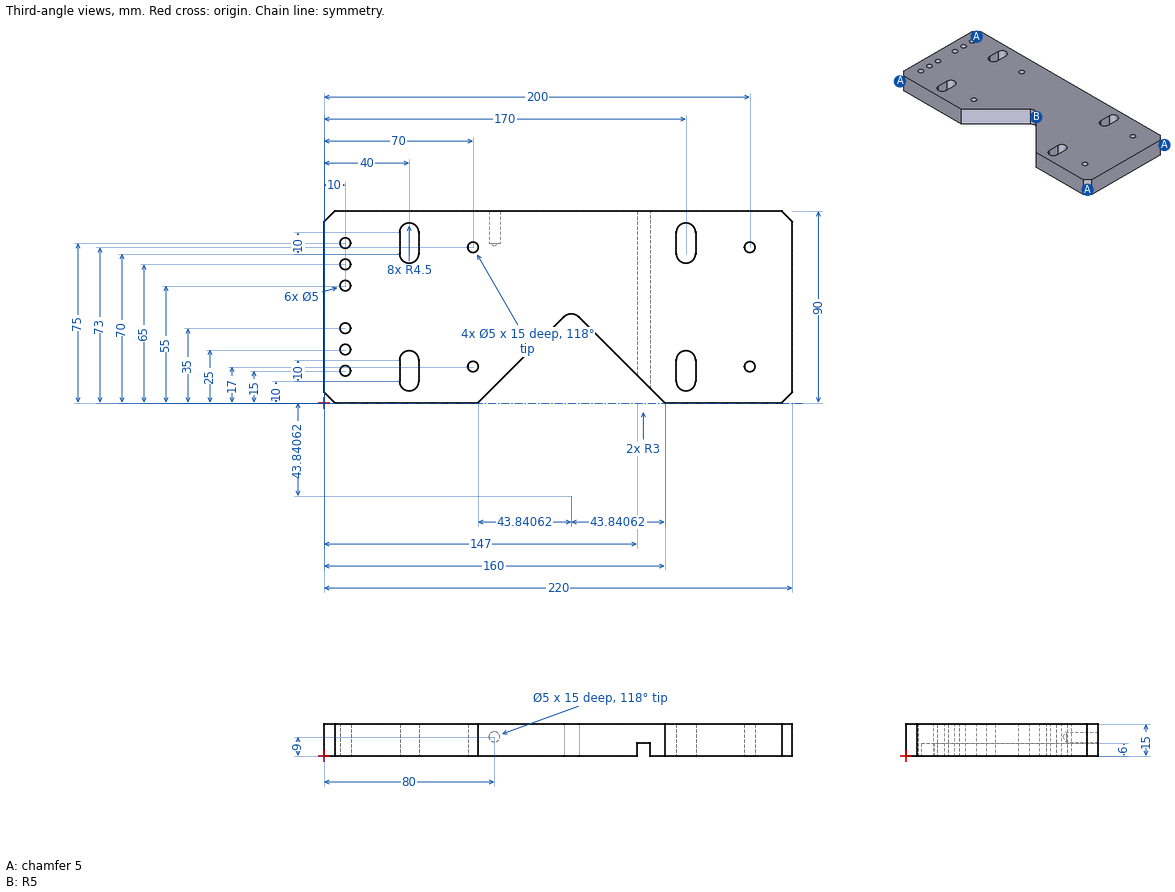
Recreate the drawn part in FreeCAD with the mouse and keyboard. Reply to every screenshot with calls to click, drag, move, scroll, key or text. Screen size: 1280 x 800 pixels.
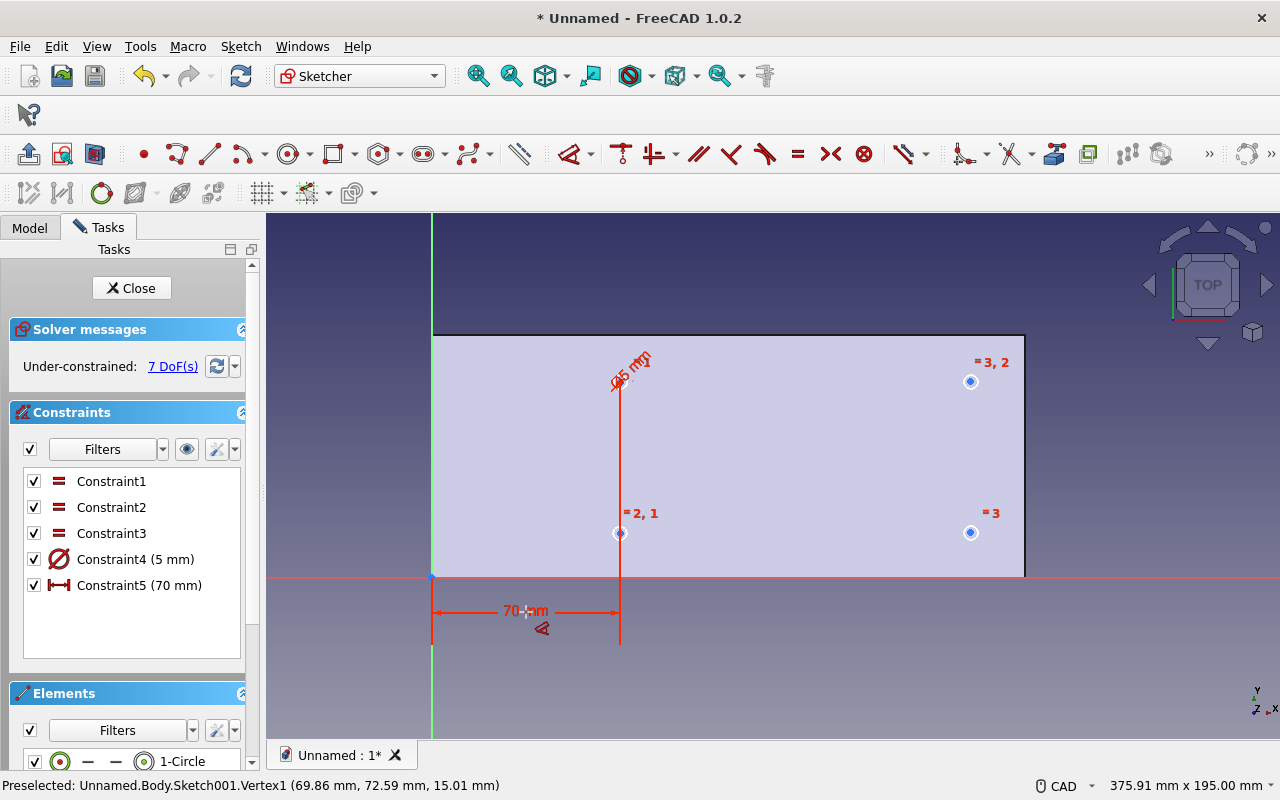
click(620, 382)
click(398, 480)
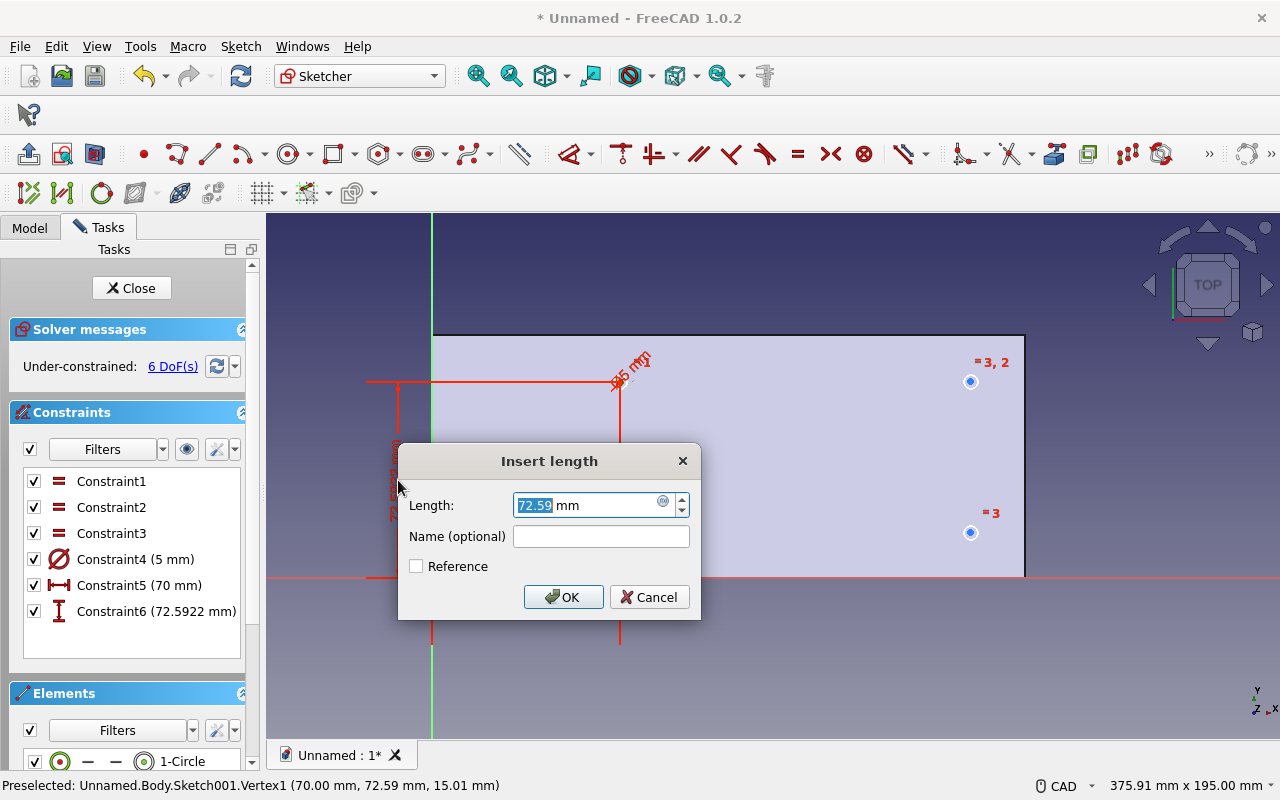
text(73)
key(Return)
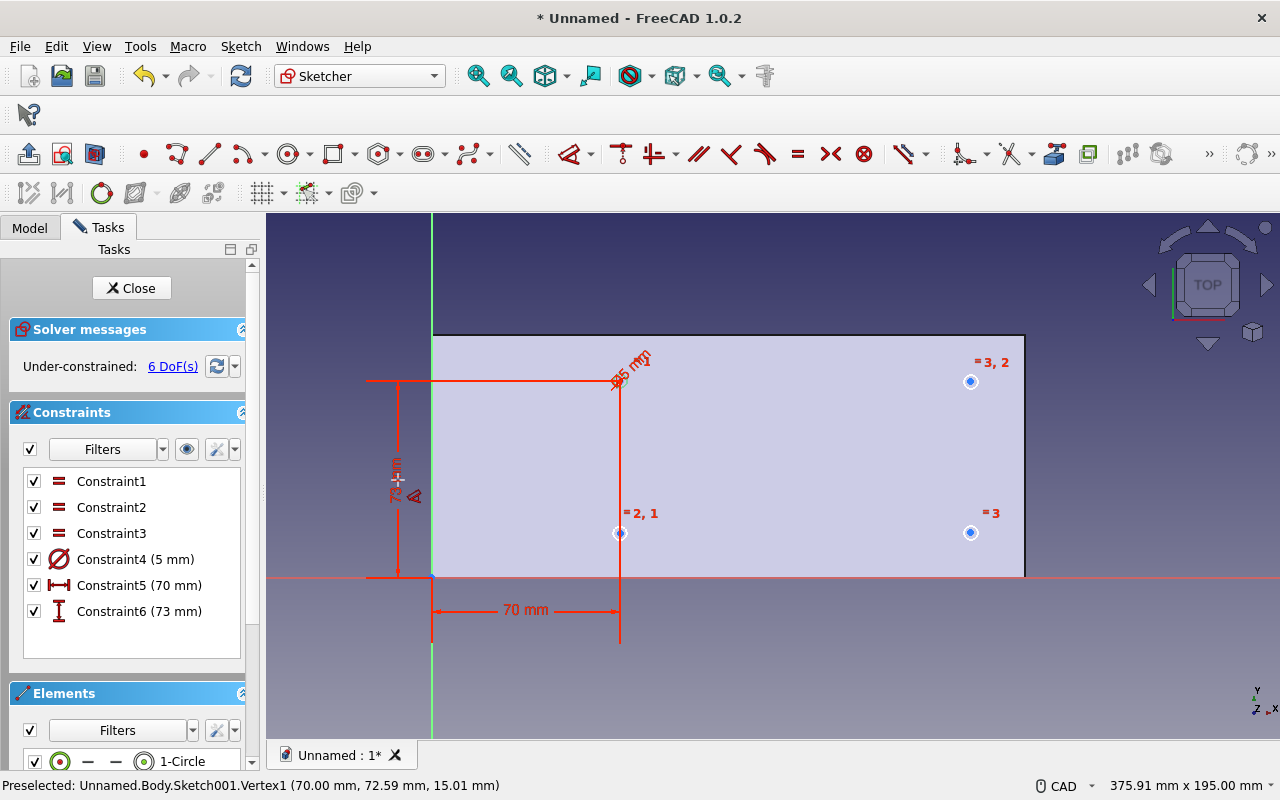
click(620, 533)
click(526, 499)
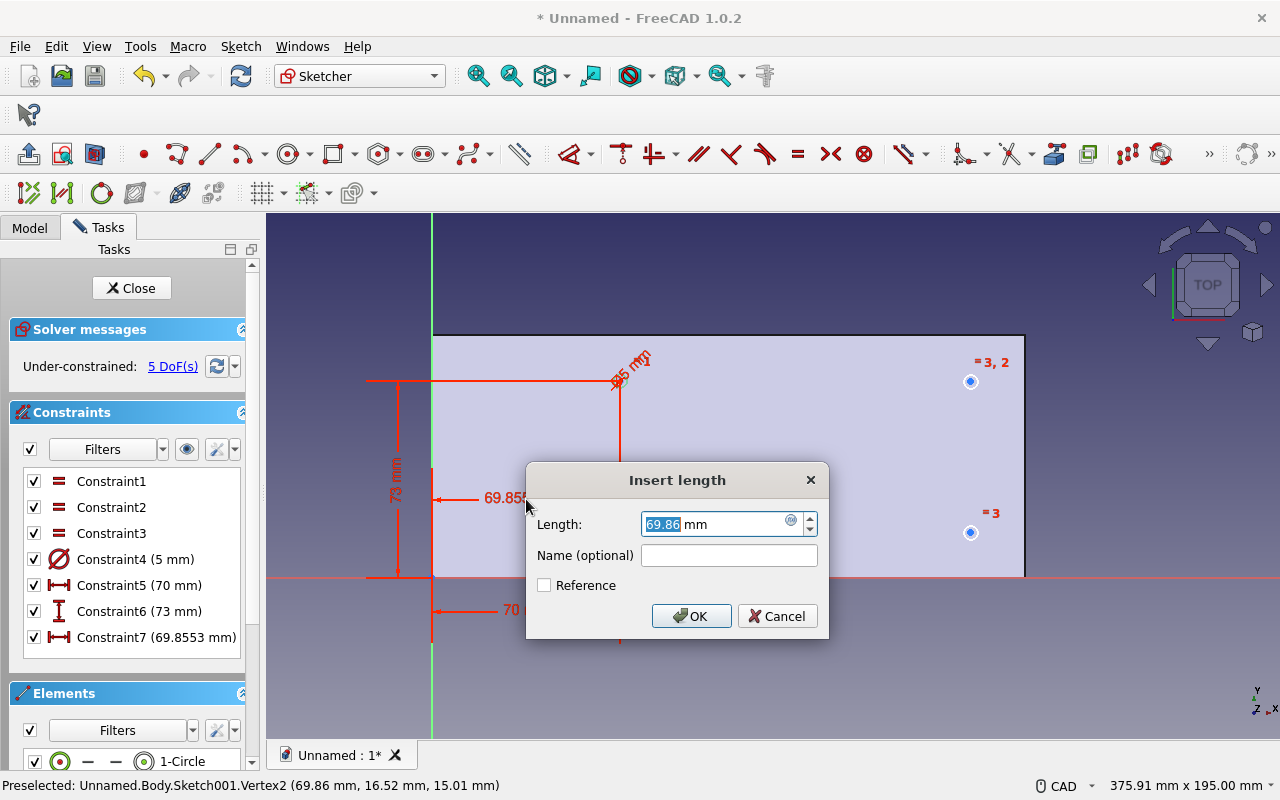
text(70)
key(Return)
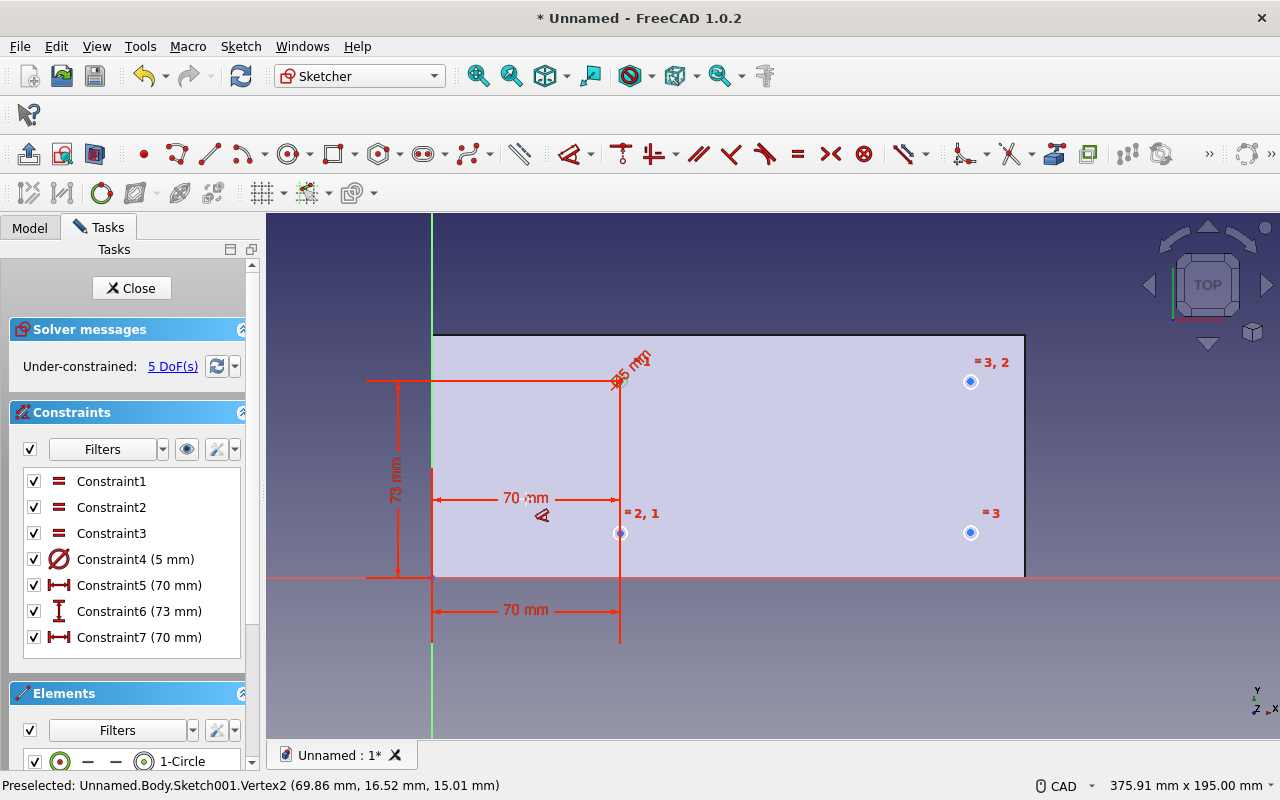
click(620, 533)
click(398, 556)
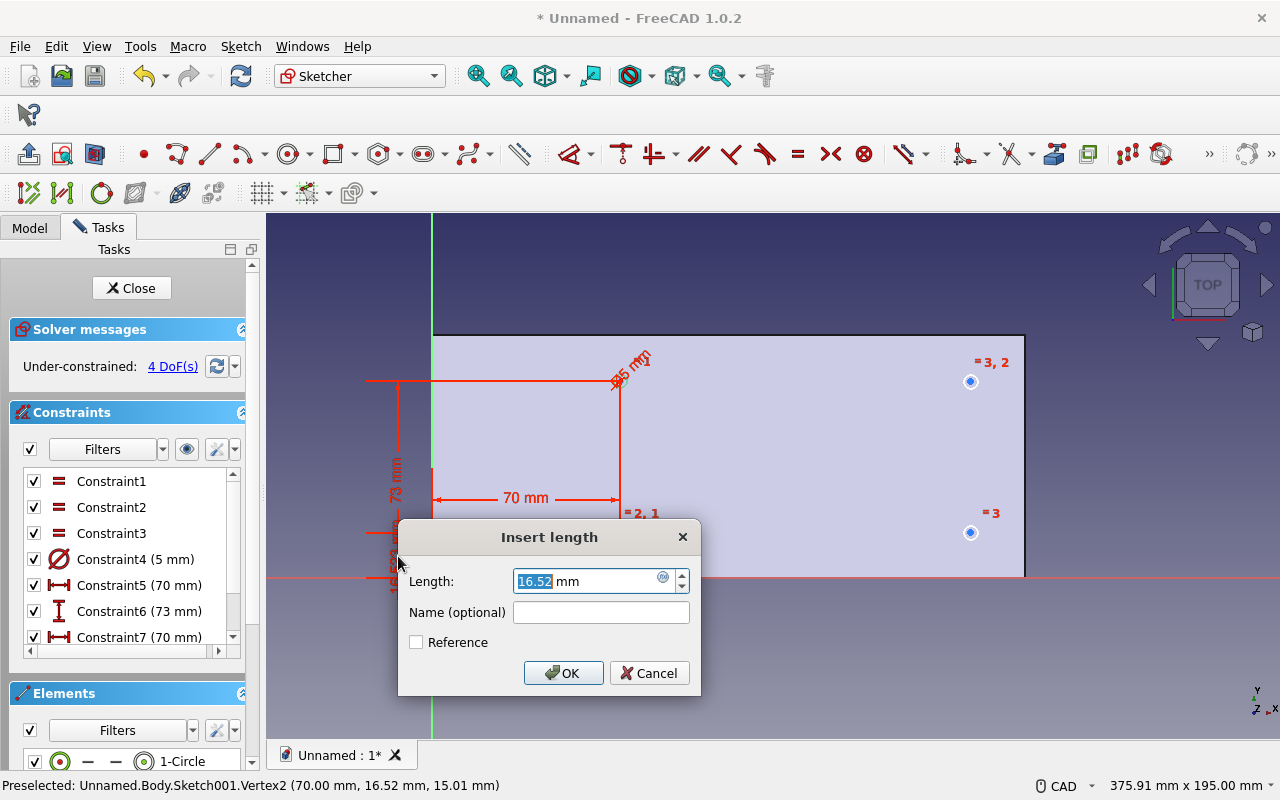
text(17)
key(Return)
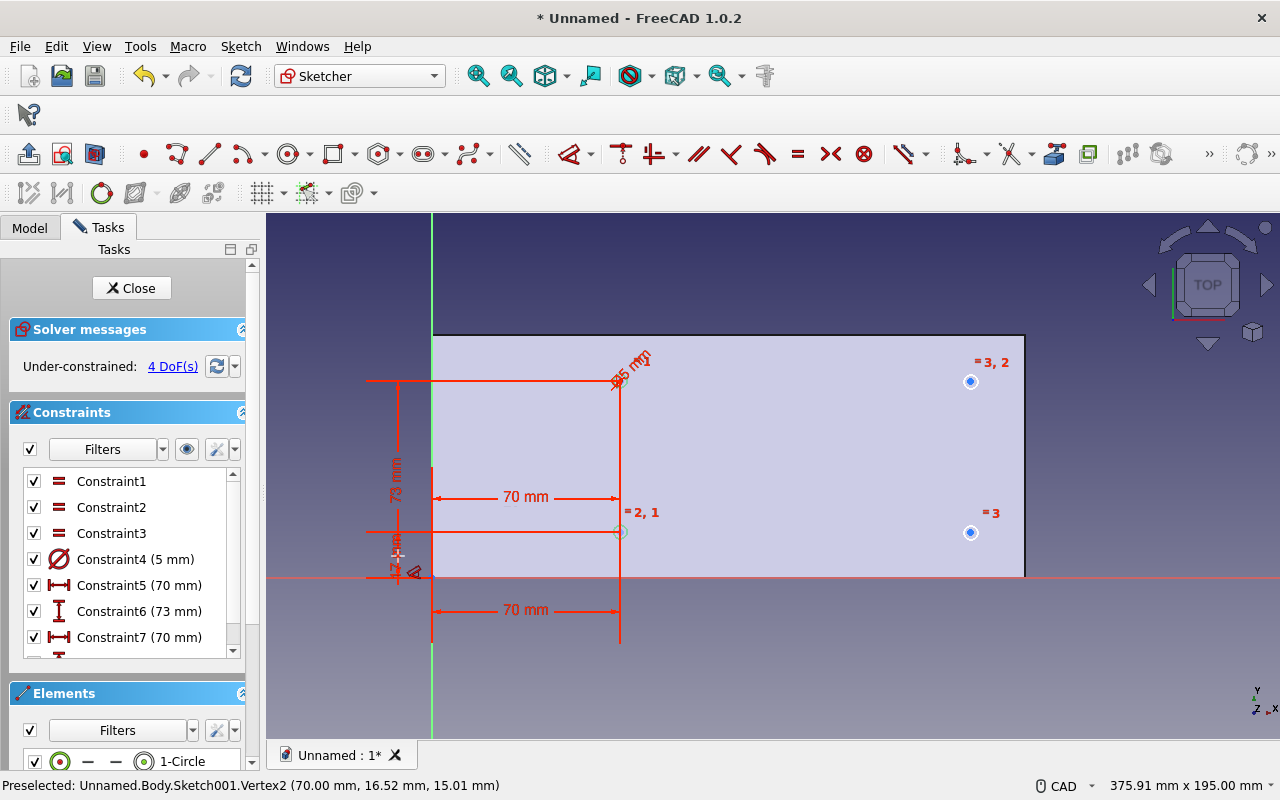
click(971, 382)
click(398, 435)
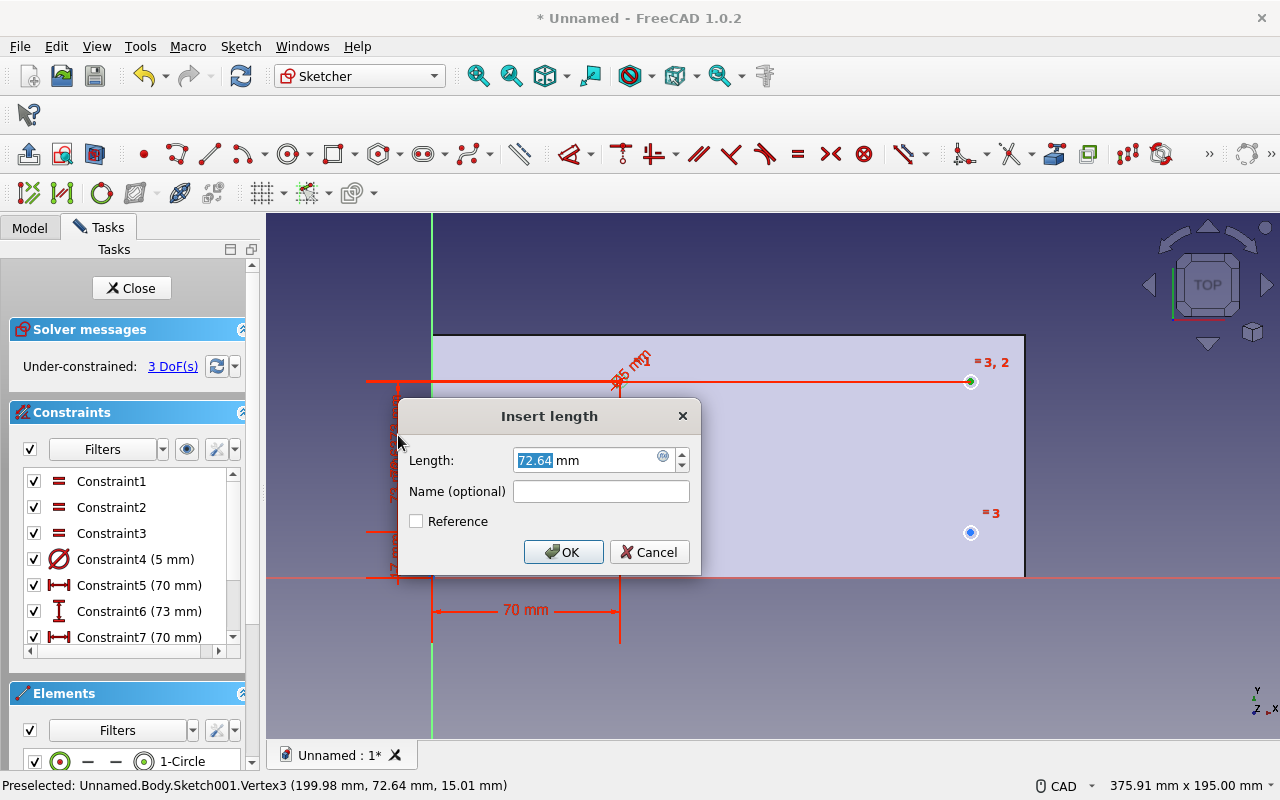
text(73)
key(Return)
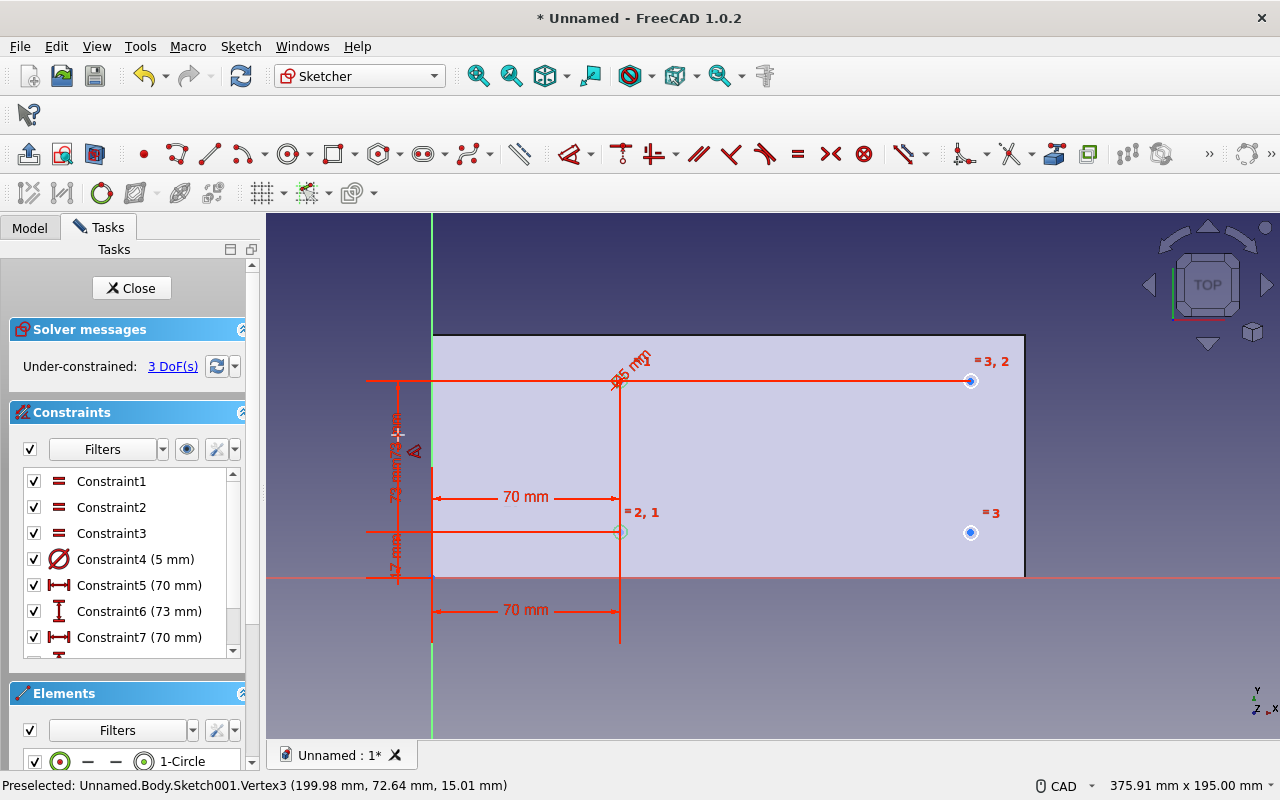
click(971, 533)
click(1005, 555)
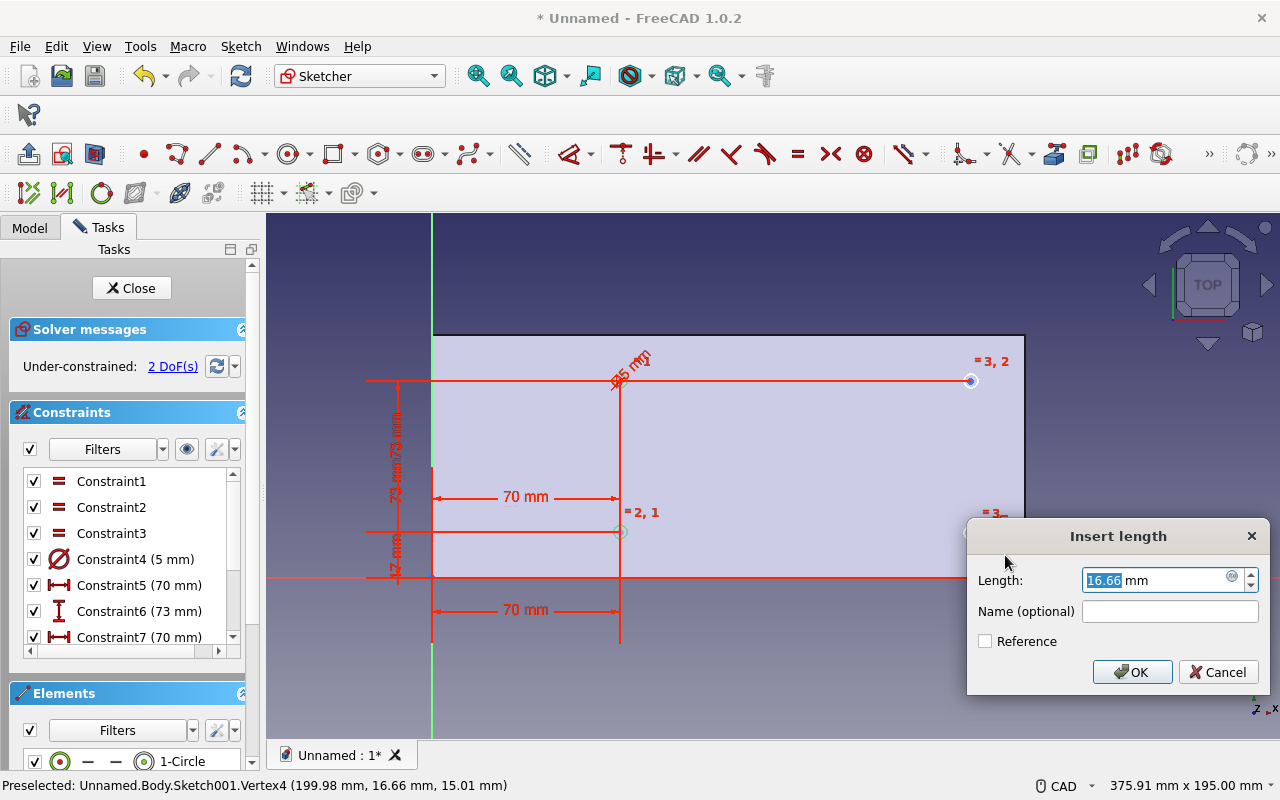
text(17)
key(Return)